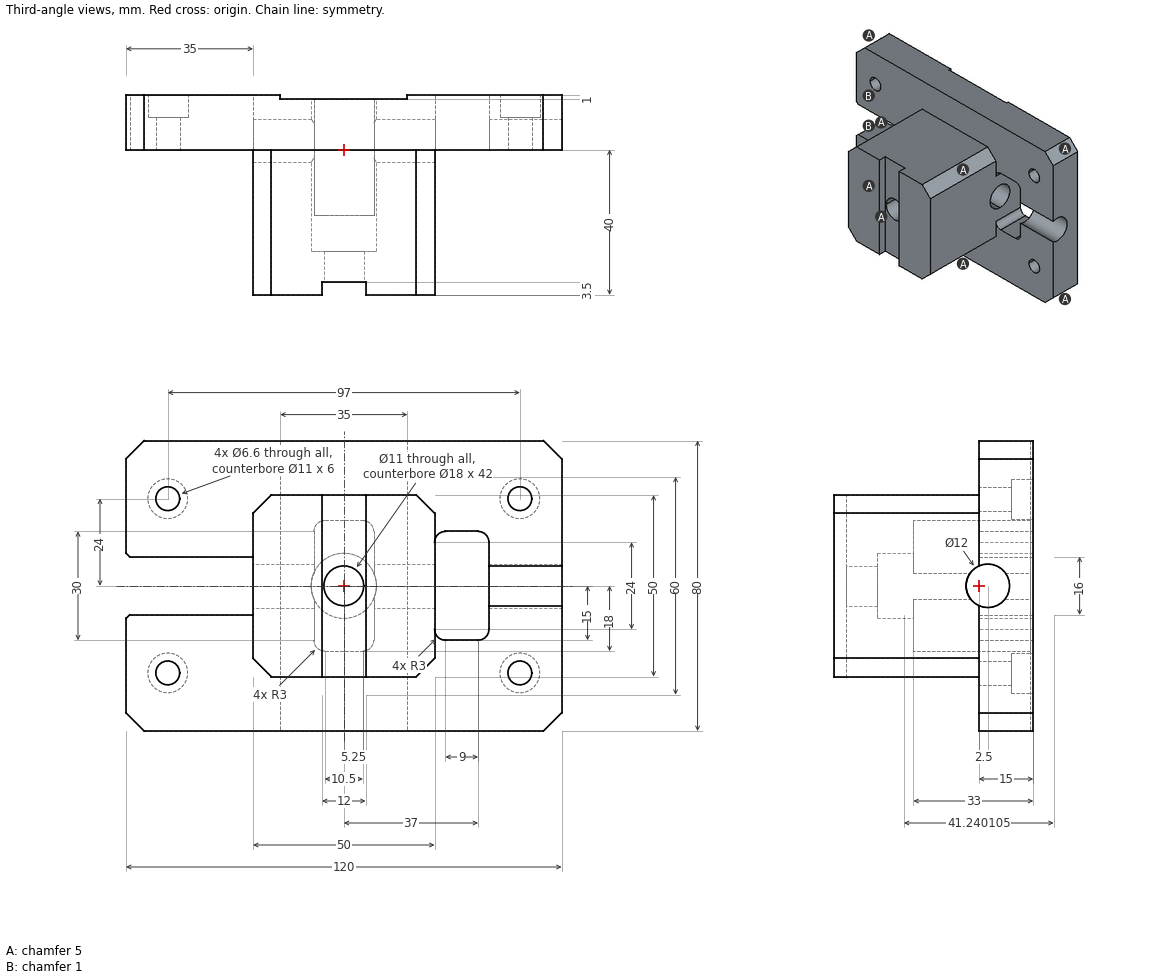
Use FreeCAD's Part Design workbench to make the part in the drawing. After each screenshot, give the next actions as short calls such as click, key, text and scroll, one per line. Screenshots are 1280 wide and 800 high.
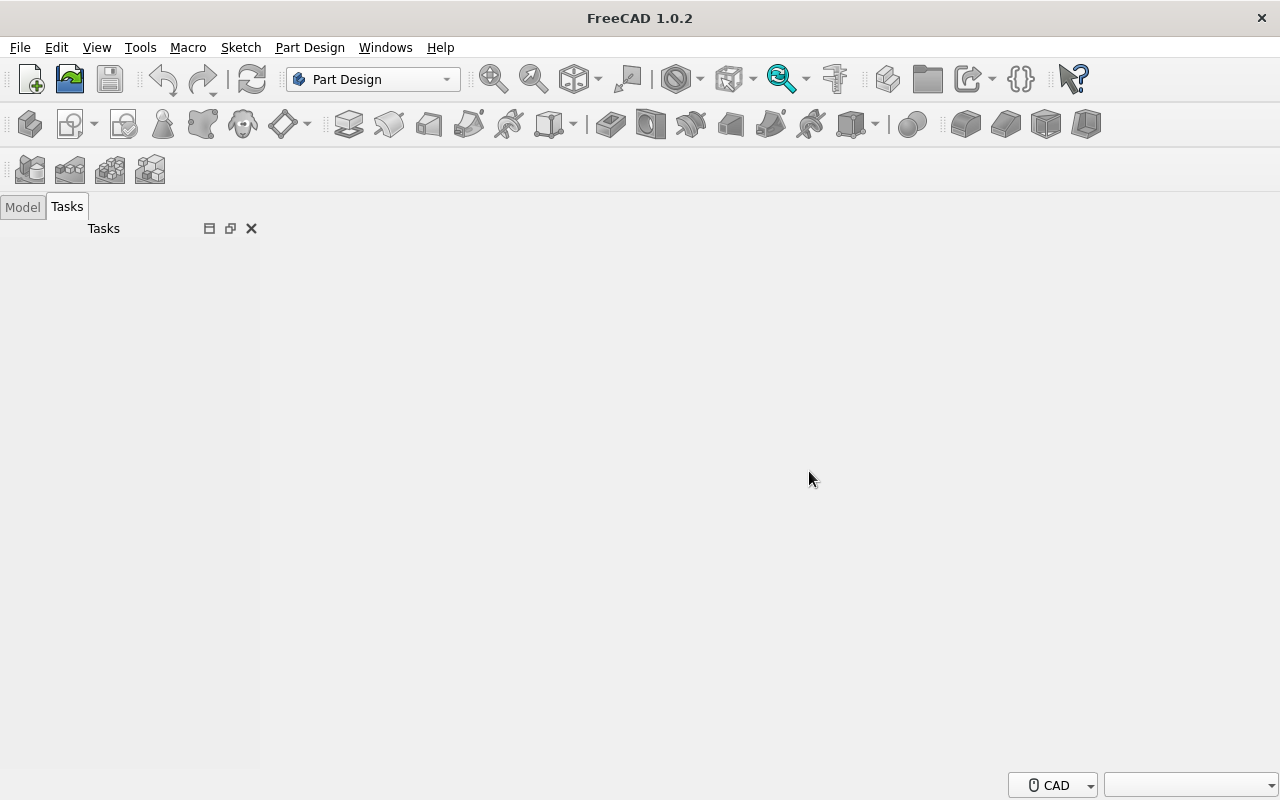
click(30, 80)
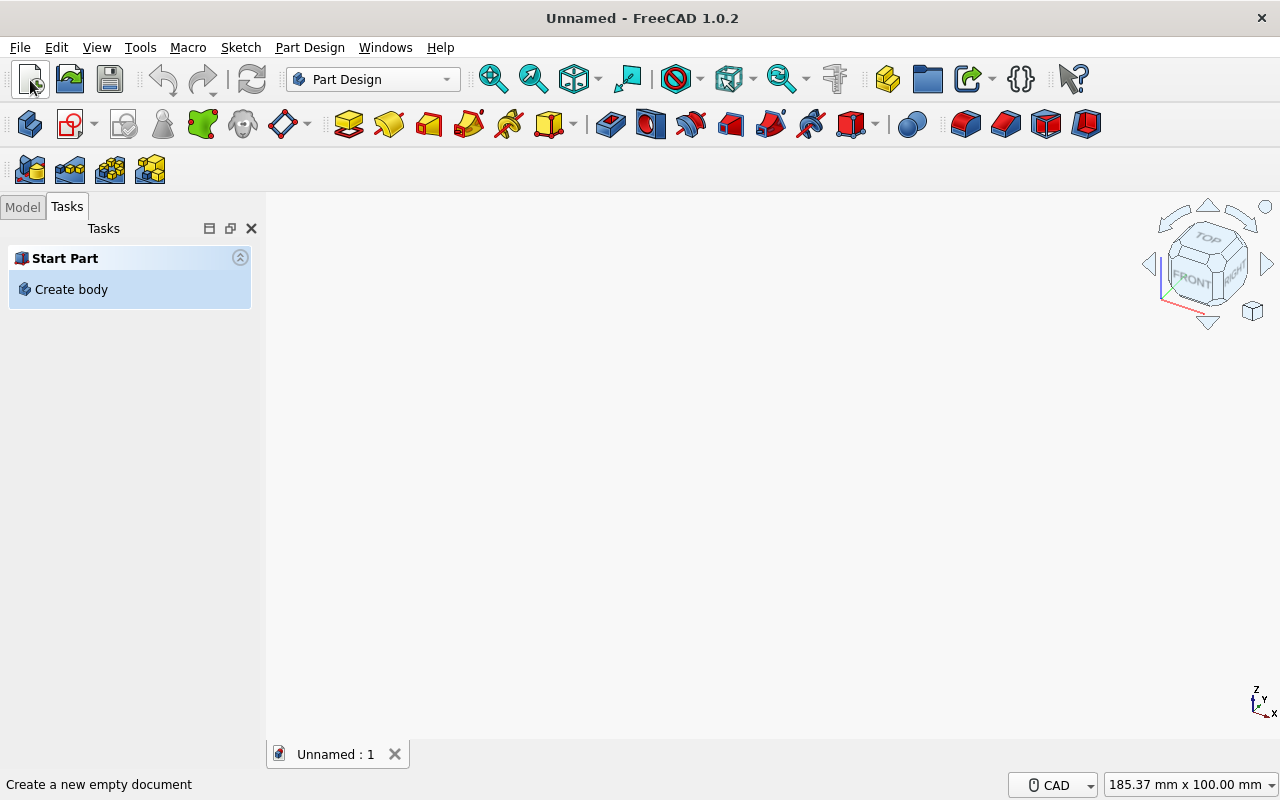
click(70, 124)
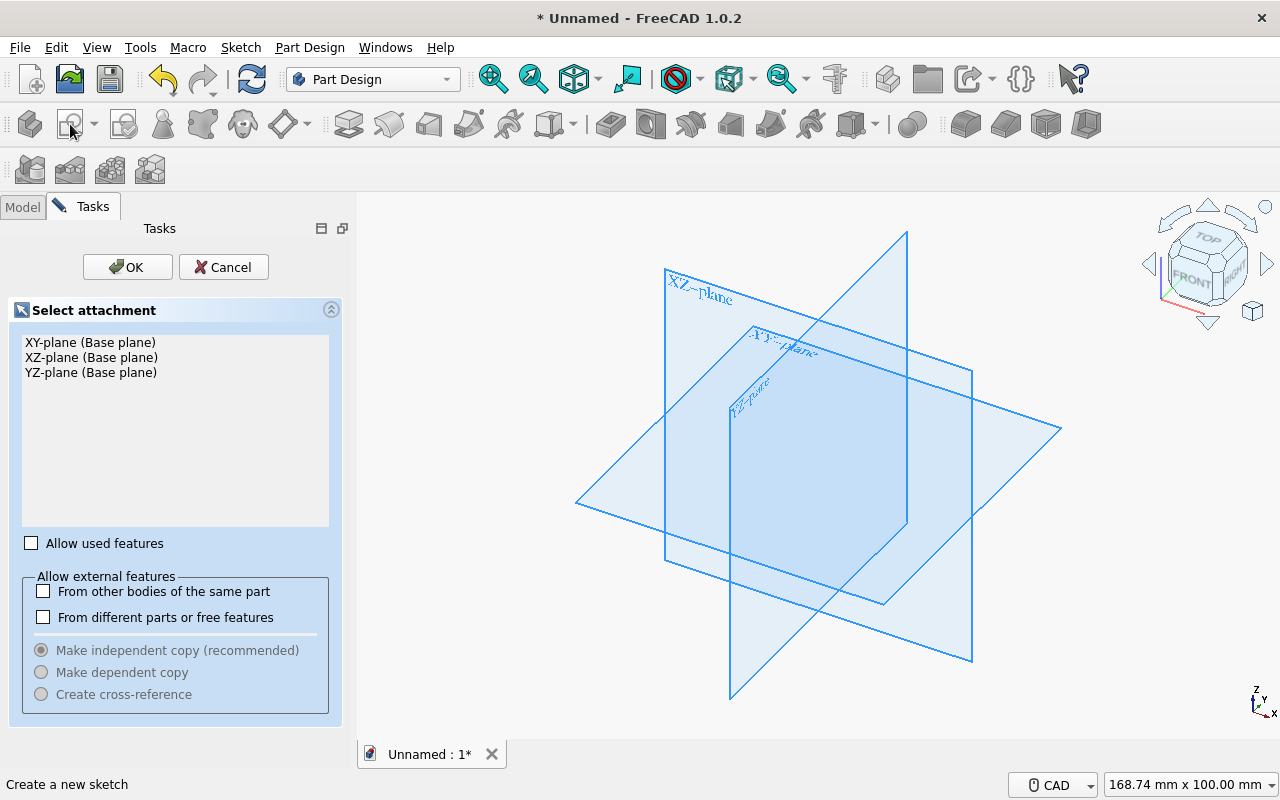
click(82, 358)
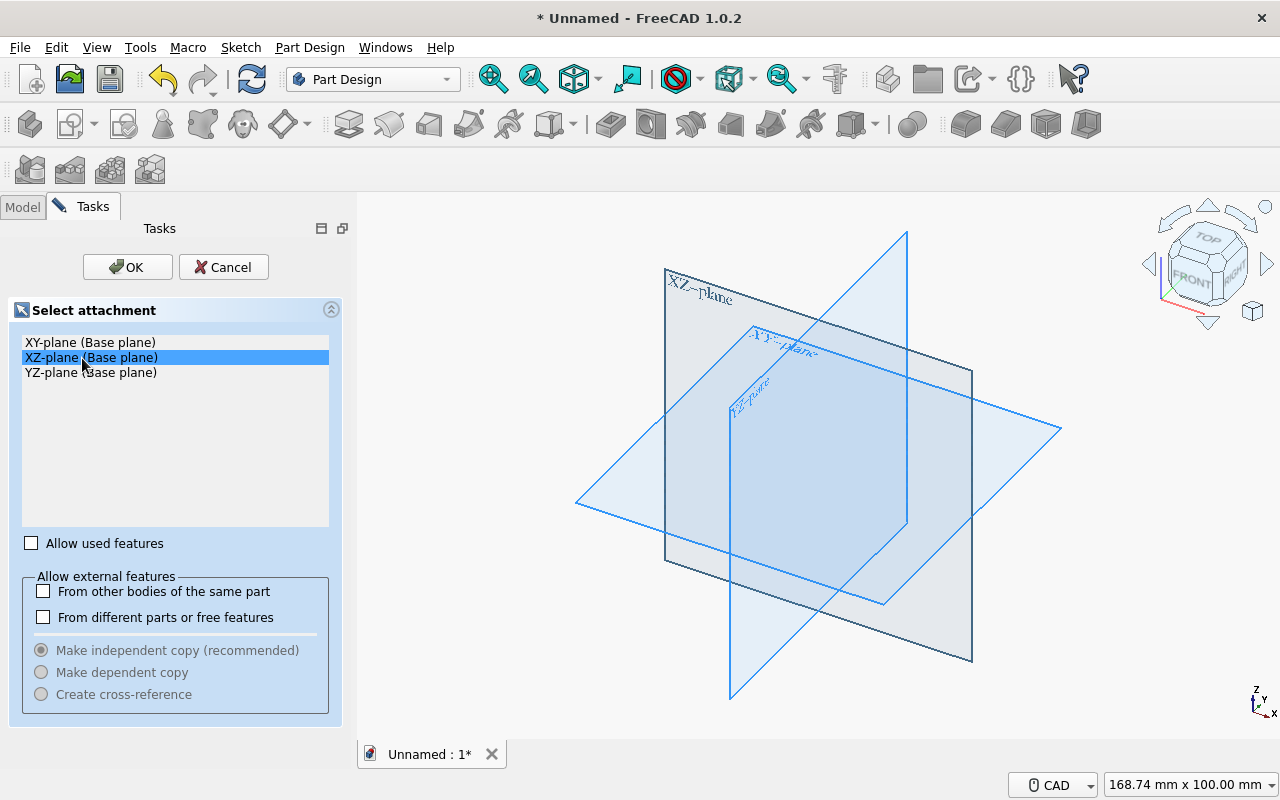
click(128, 267)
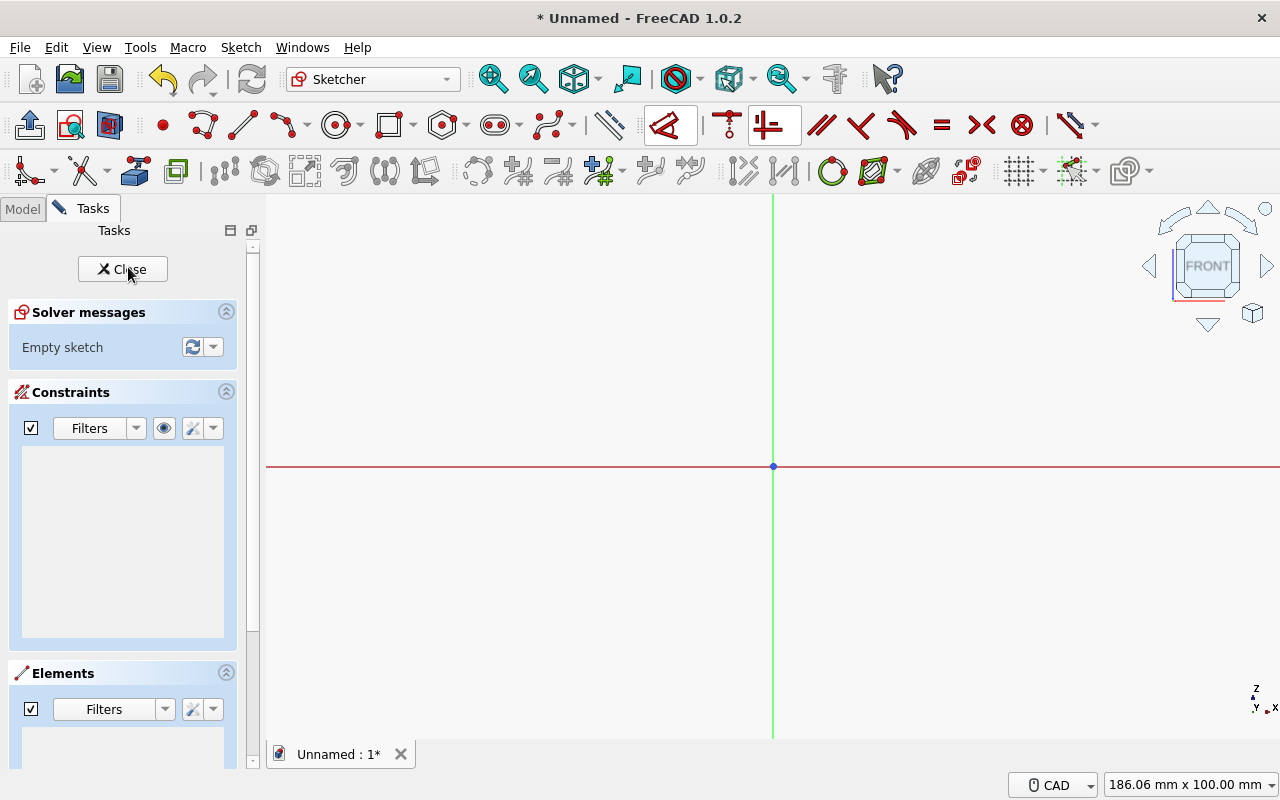
scroll(395, 467, down, 1)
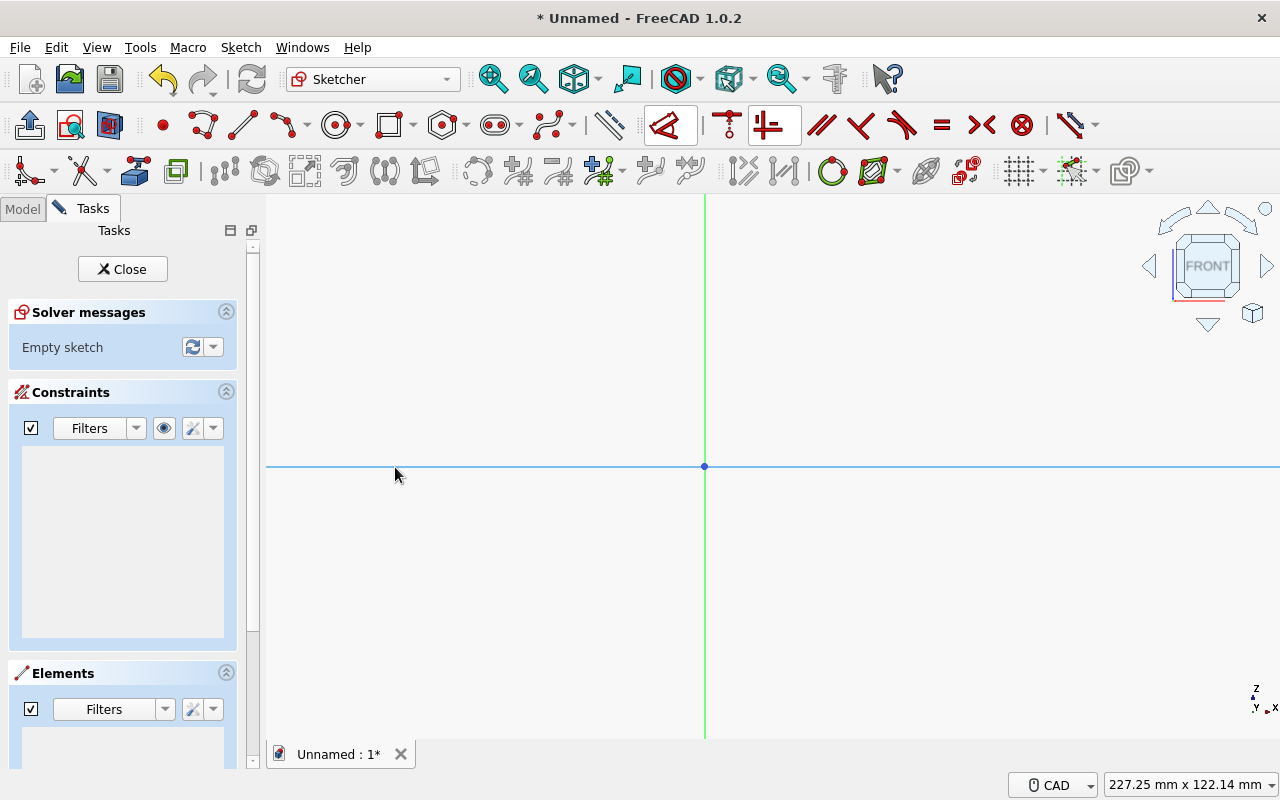
click(416, 126)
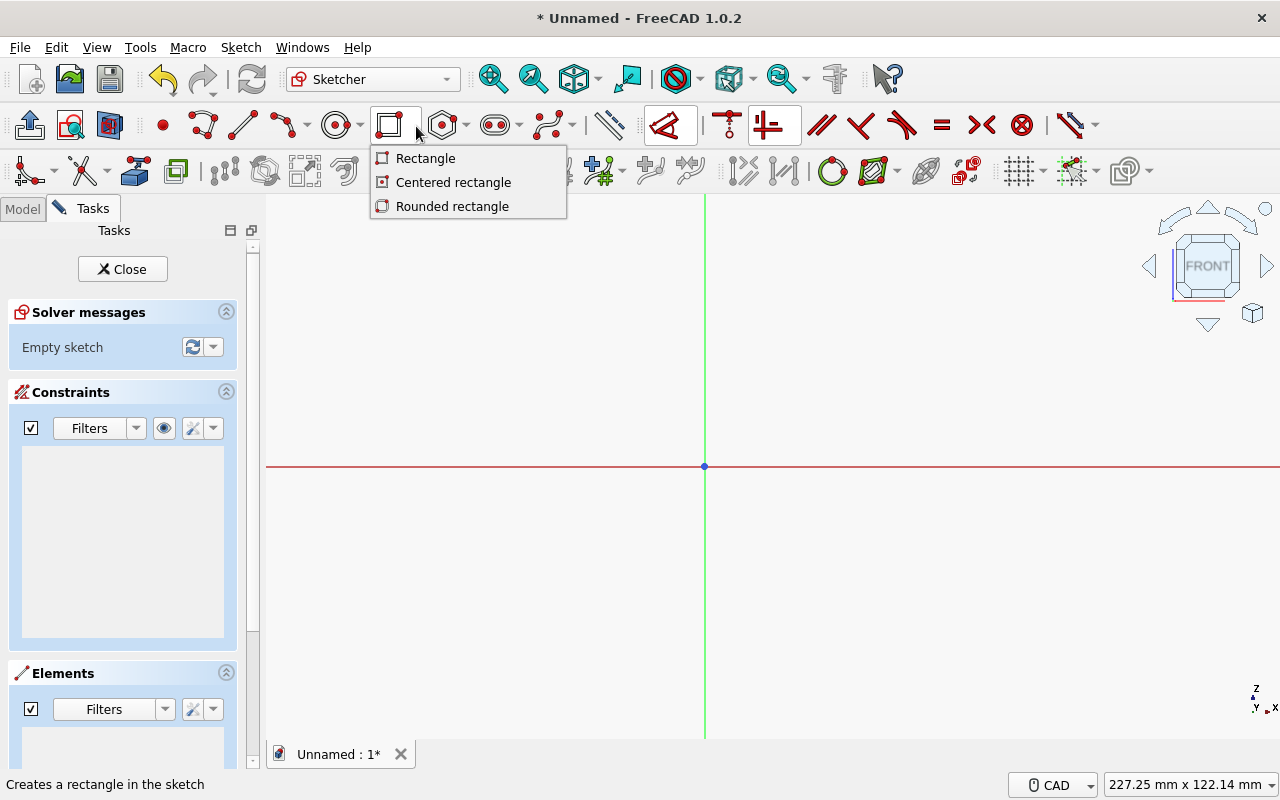
click(468, 182)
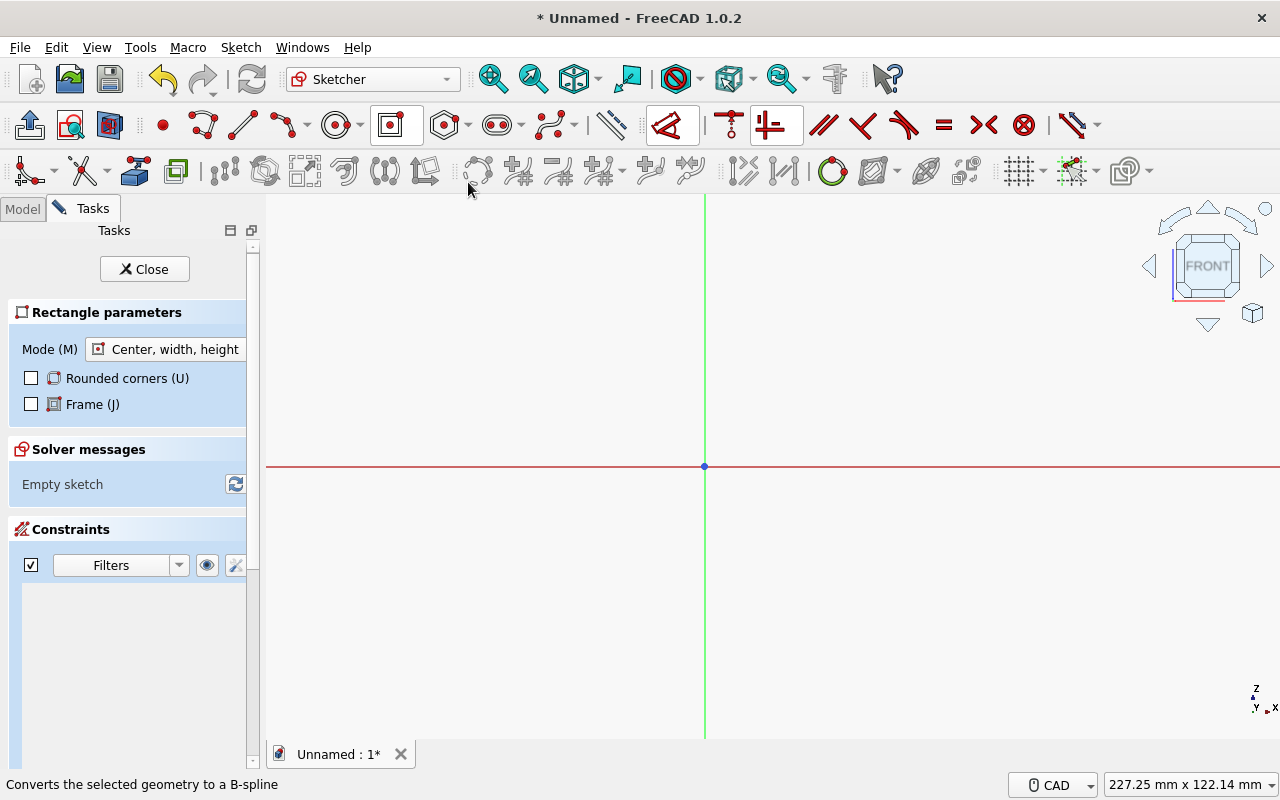
click(705, 467)
click(972, 288)
key(Escape)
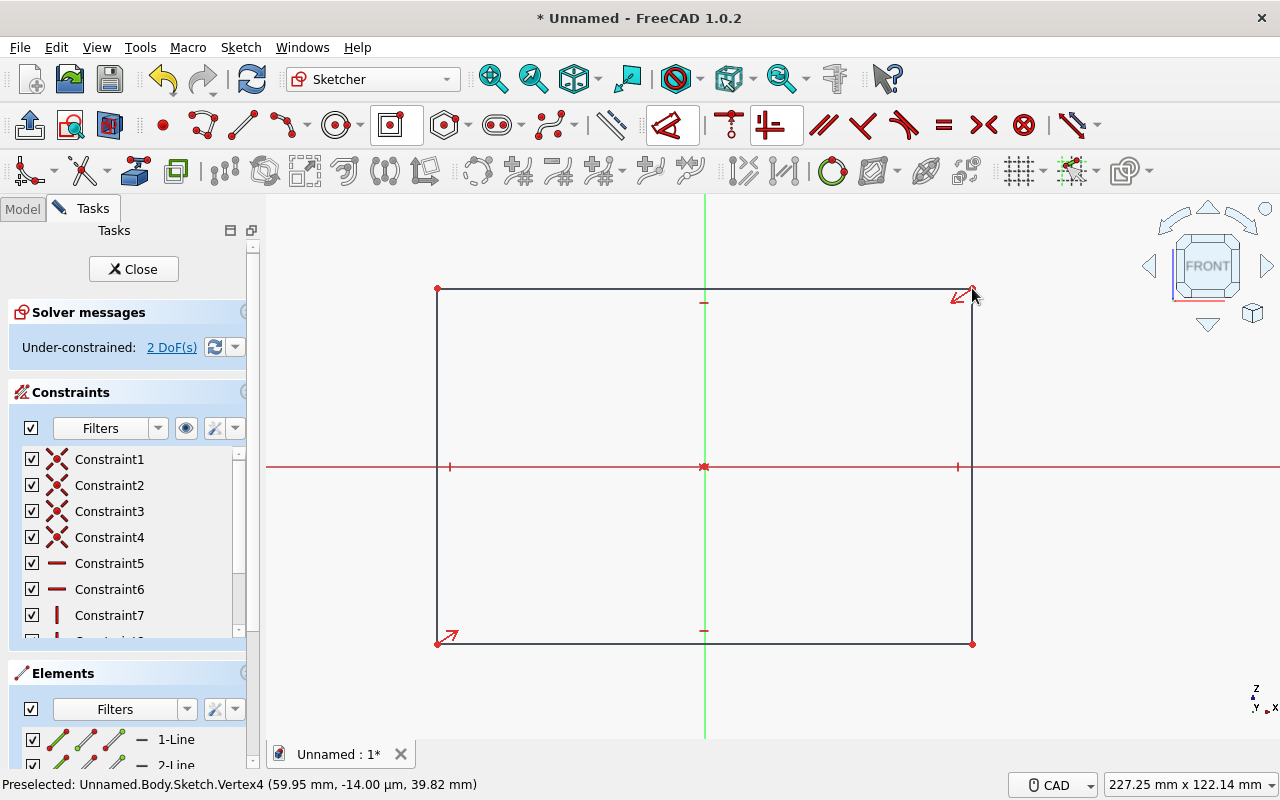
click(972, 538)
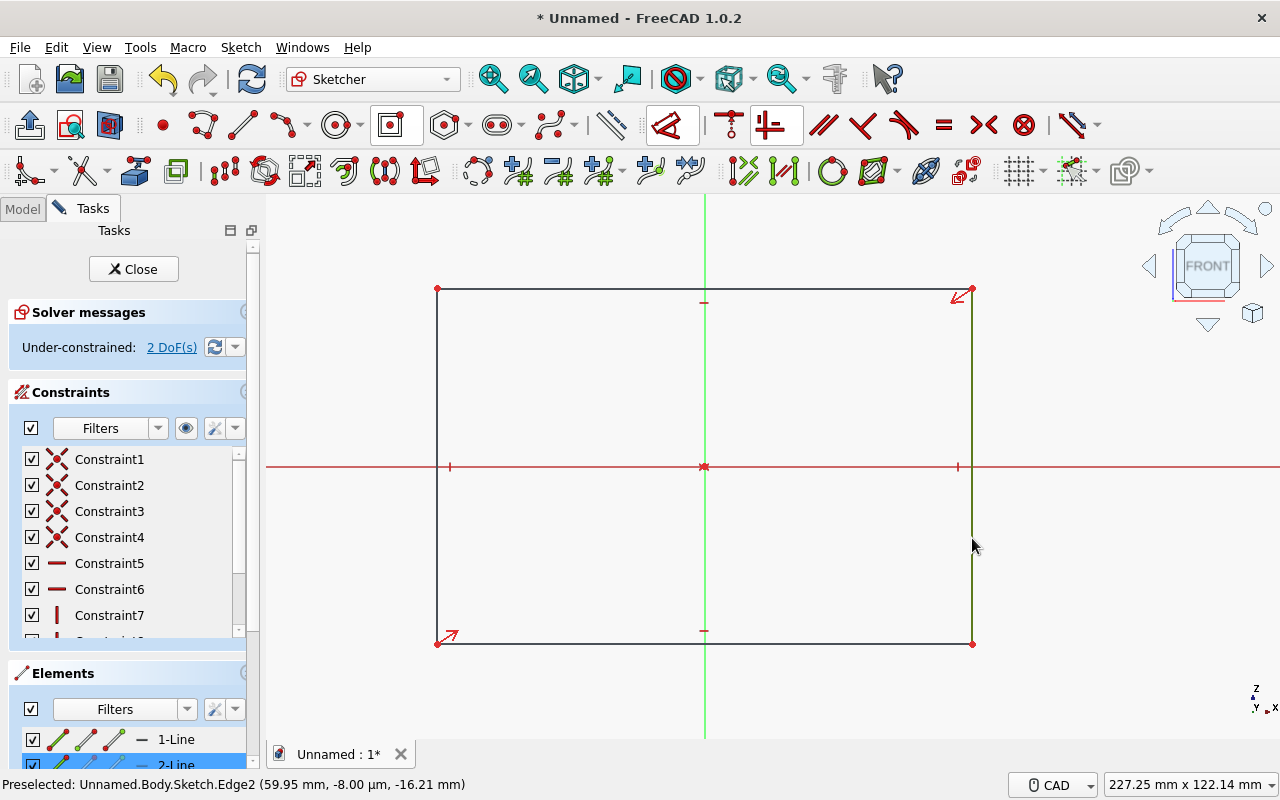
click(694, 126)